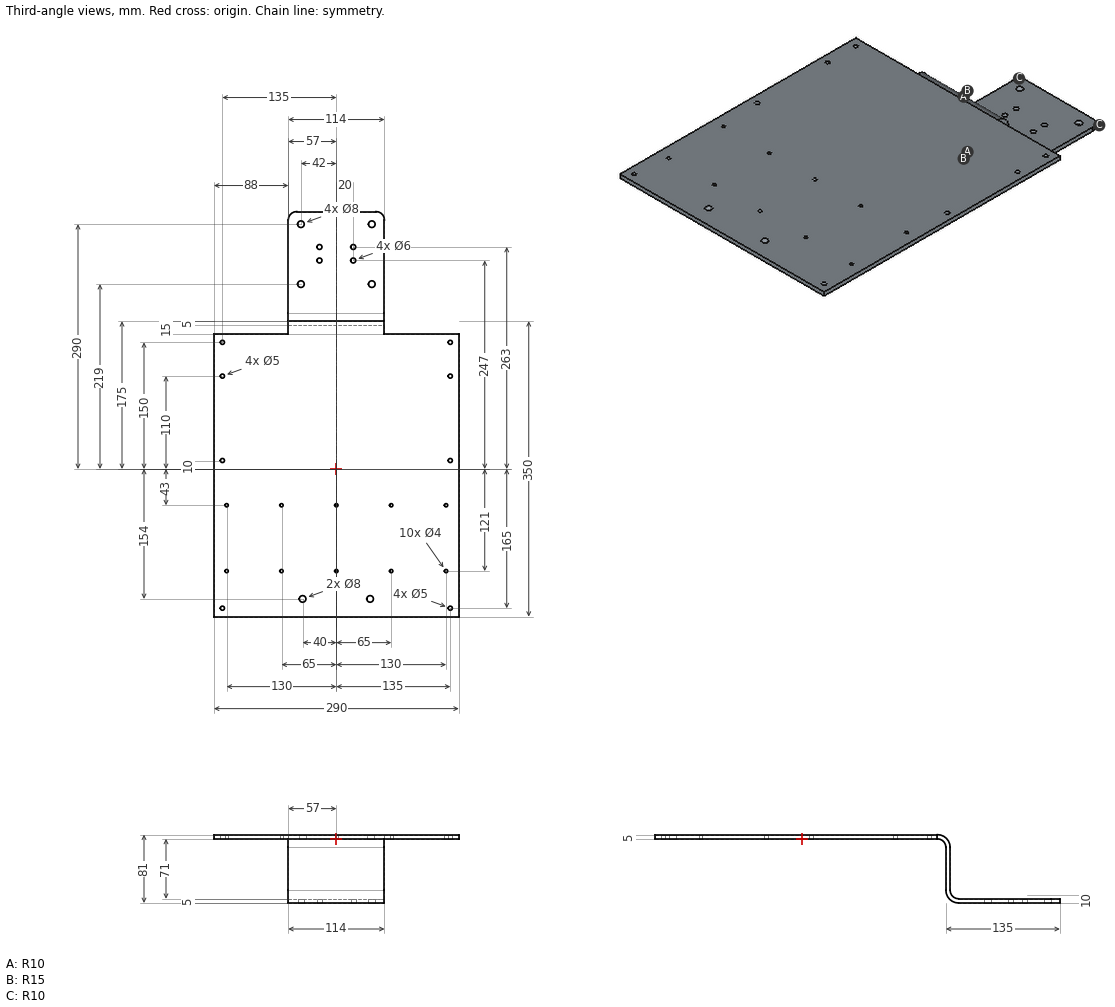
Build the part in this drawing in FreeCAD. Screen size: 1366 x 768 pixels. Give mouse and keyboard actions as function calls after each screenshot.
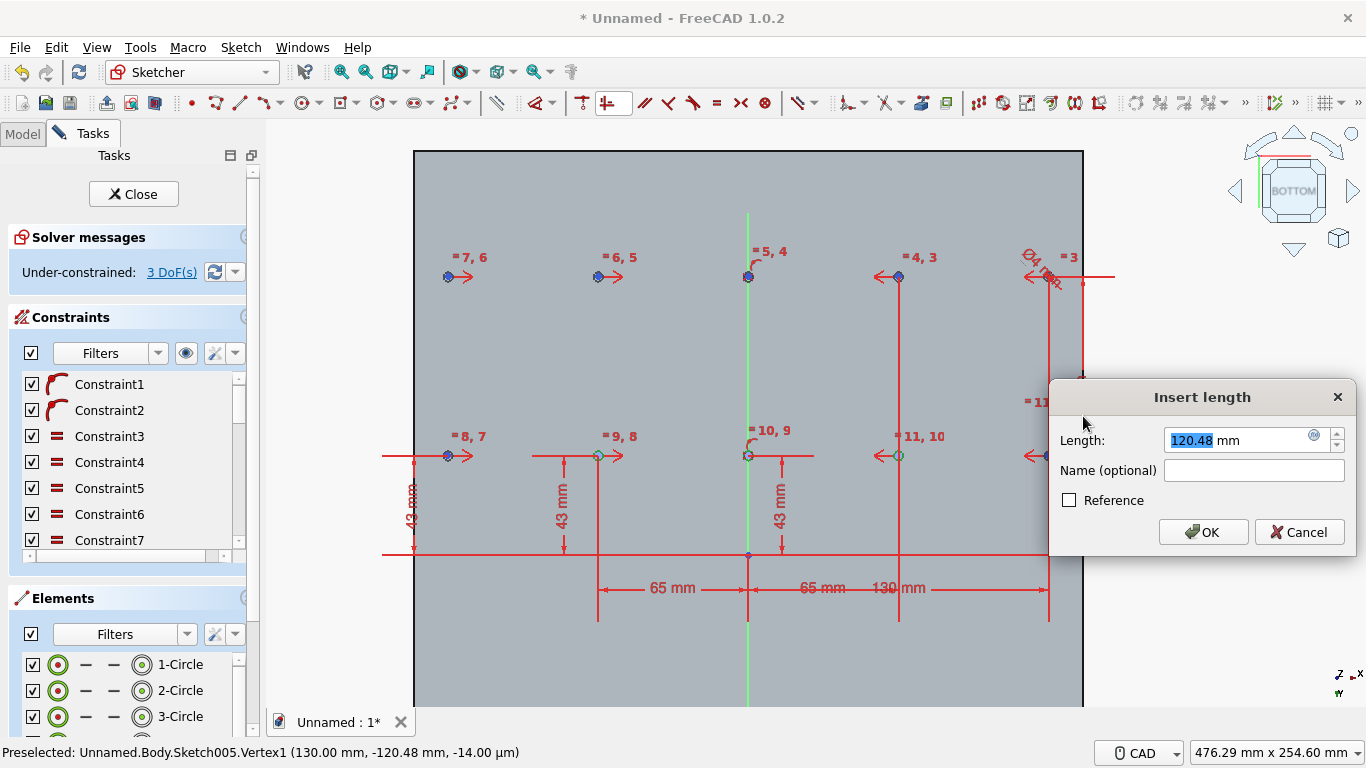
text(121)
key(Return)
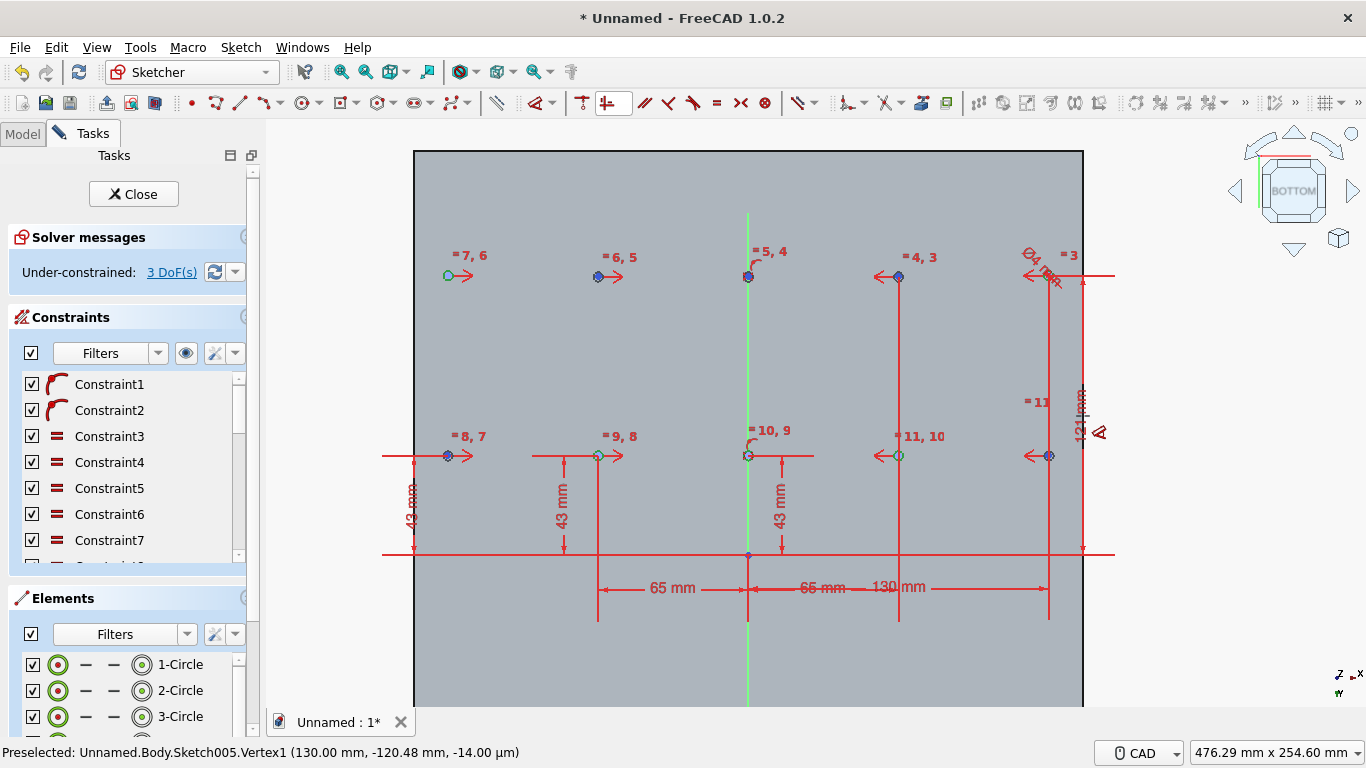
click(899, 277)
click(933, 416)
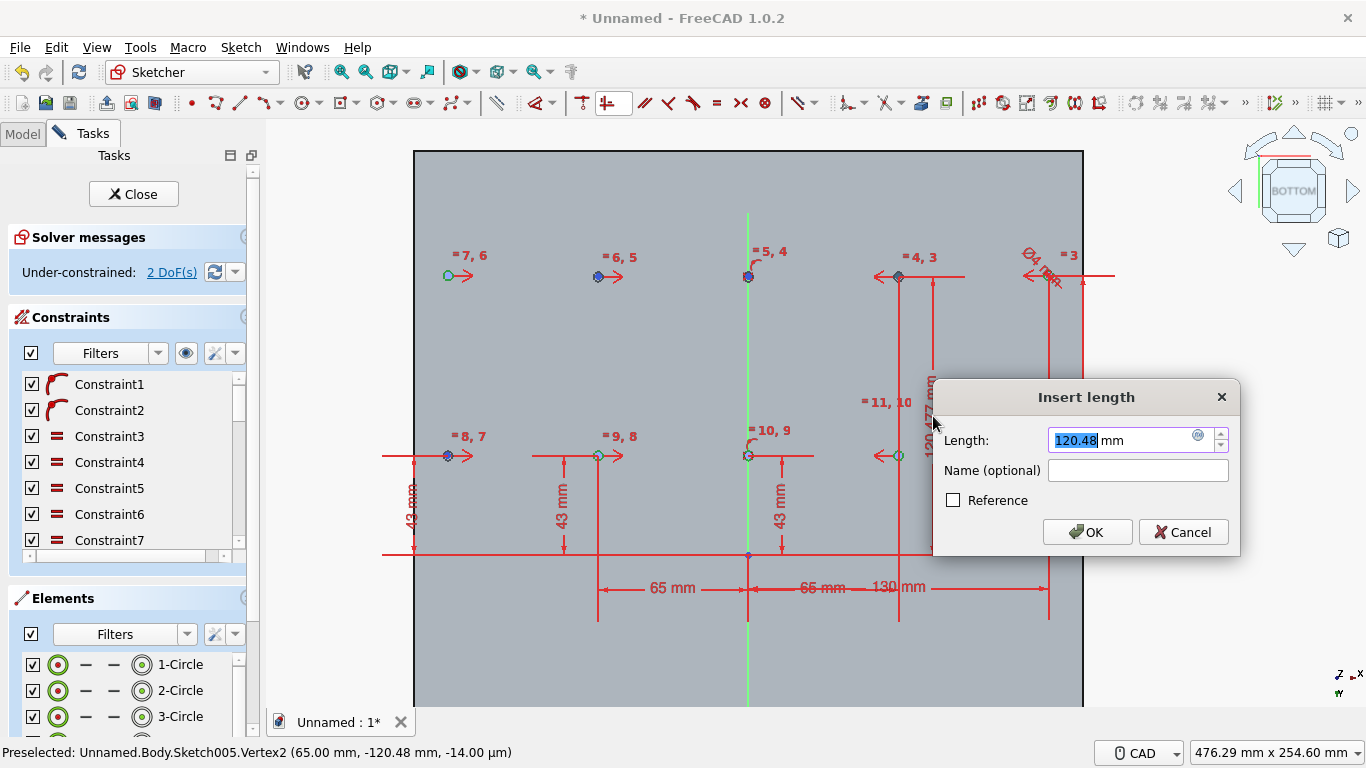
text(121)
key(Return)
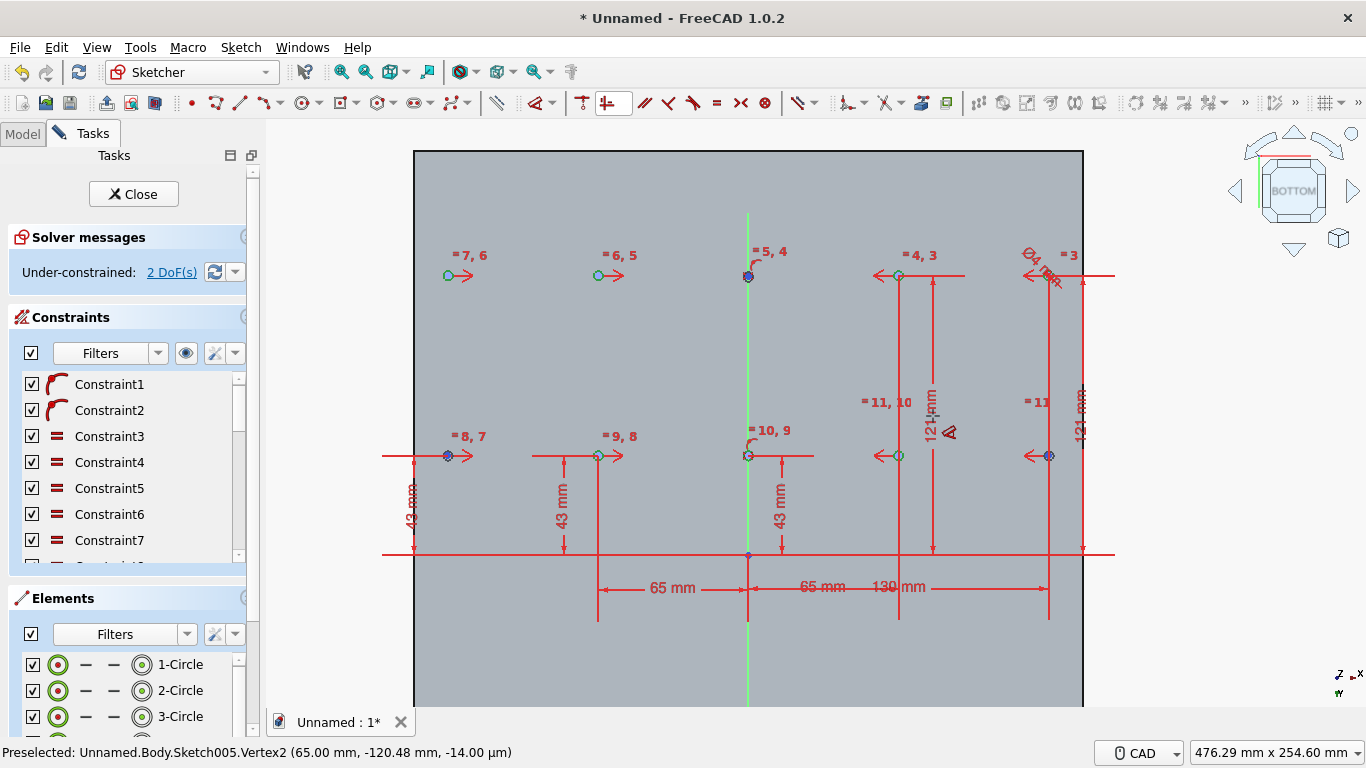
click(748, 277)
click(782, 416)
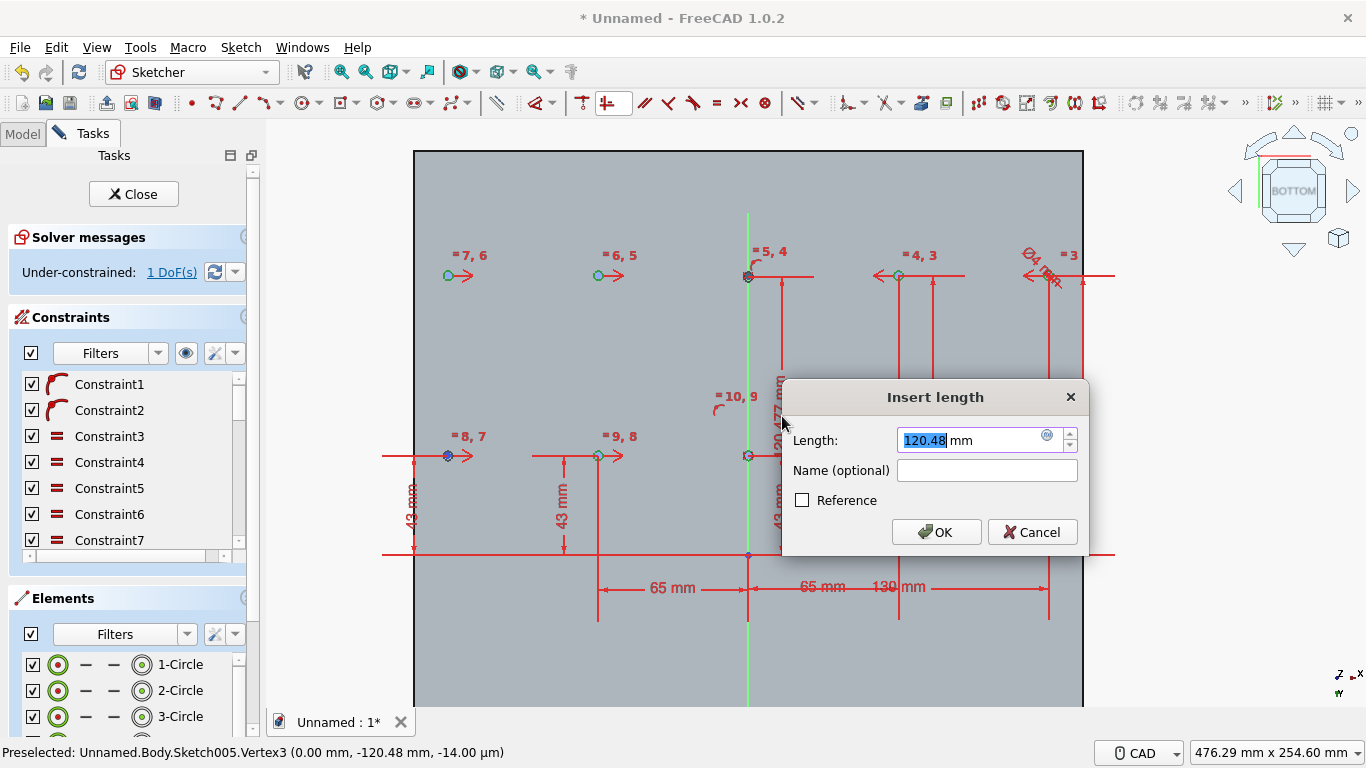
text(121)
key(Return)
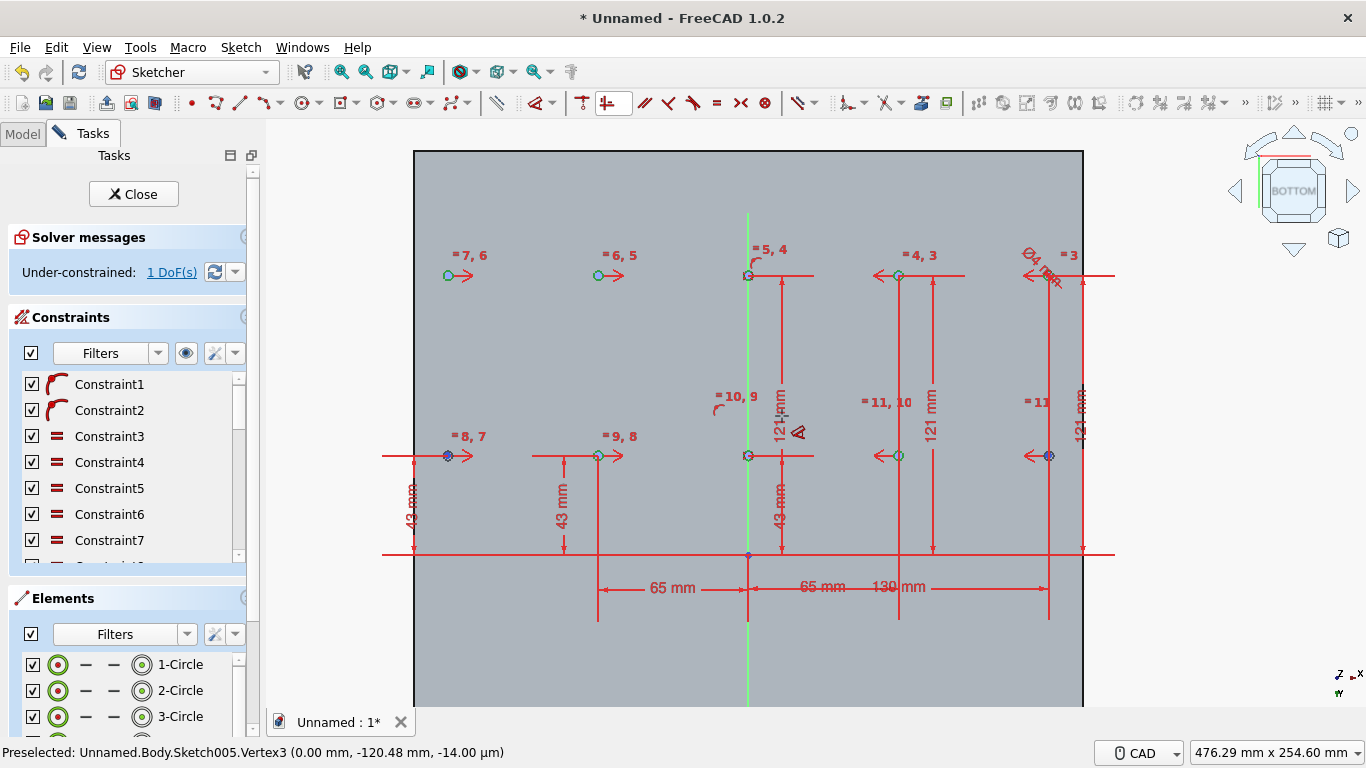
click(448, 456)
click(598, 589)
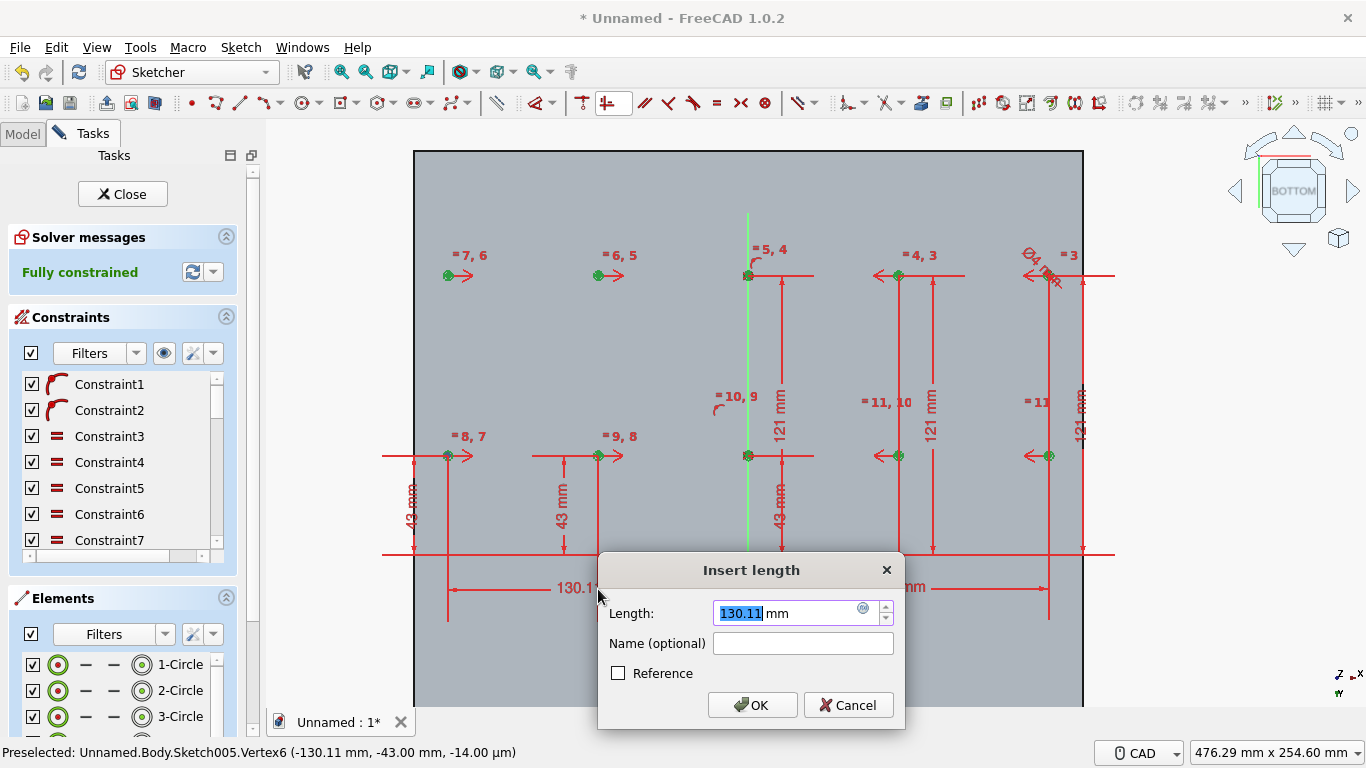
text(130)
key(Return)
key(Escape)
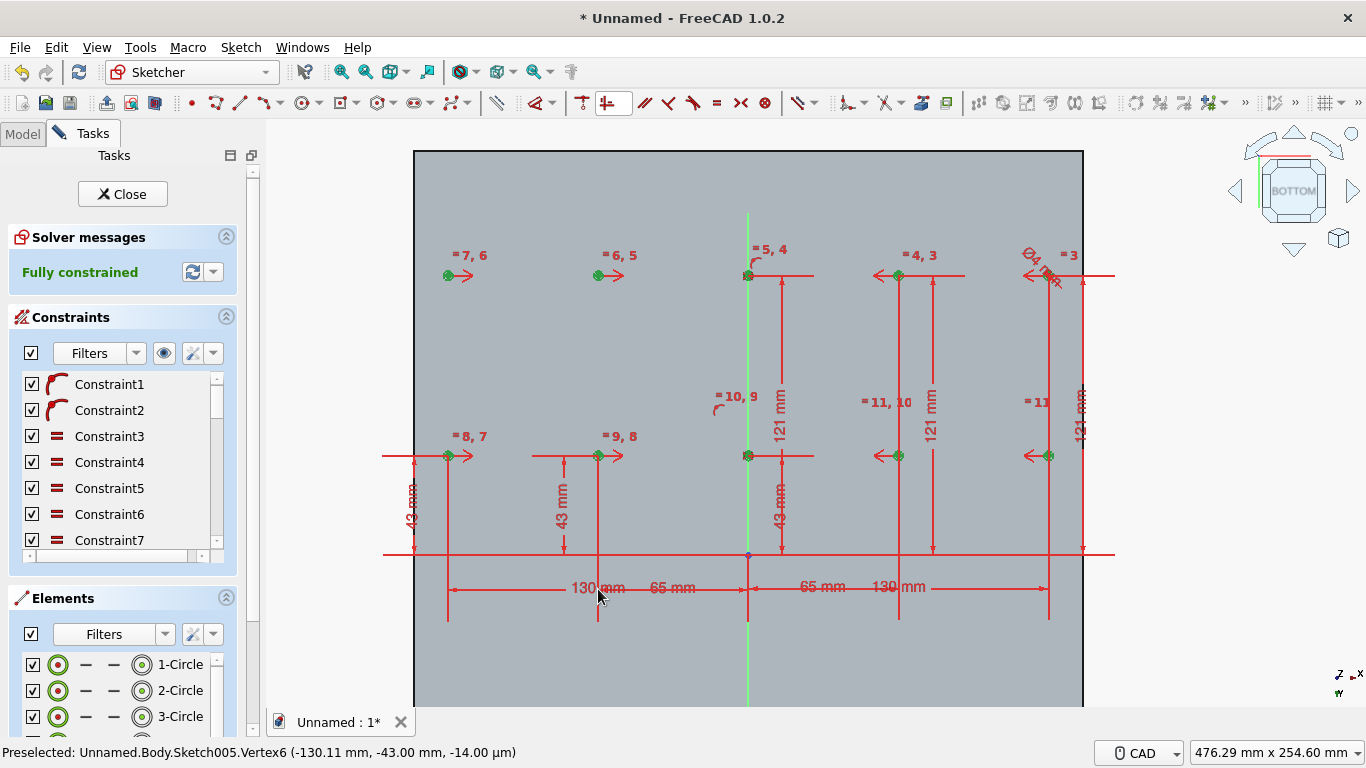
click(123, 194)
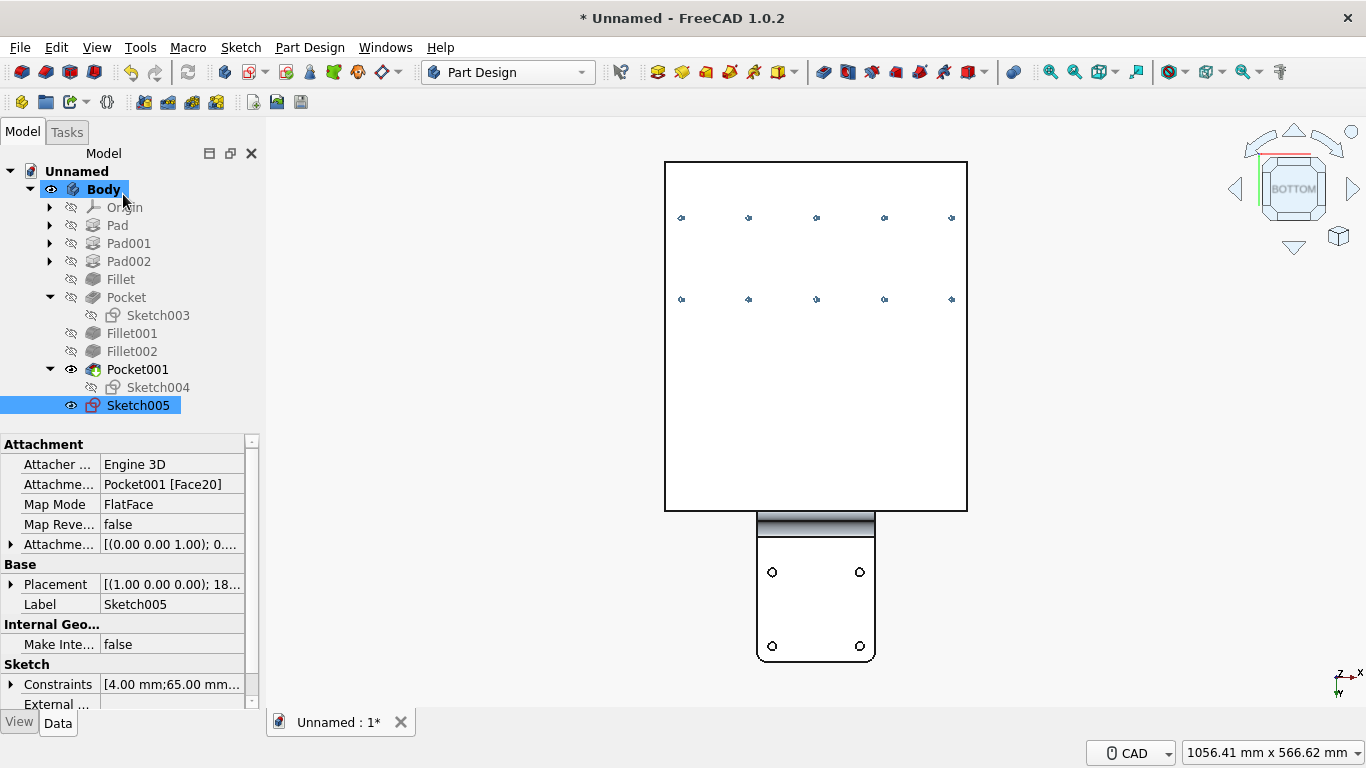
click(824, 72)